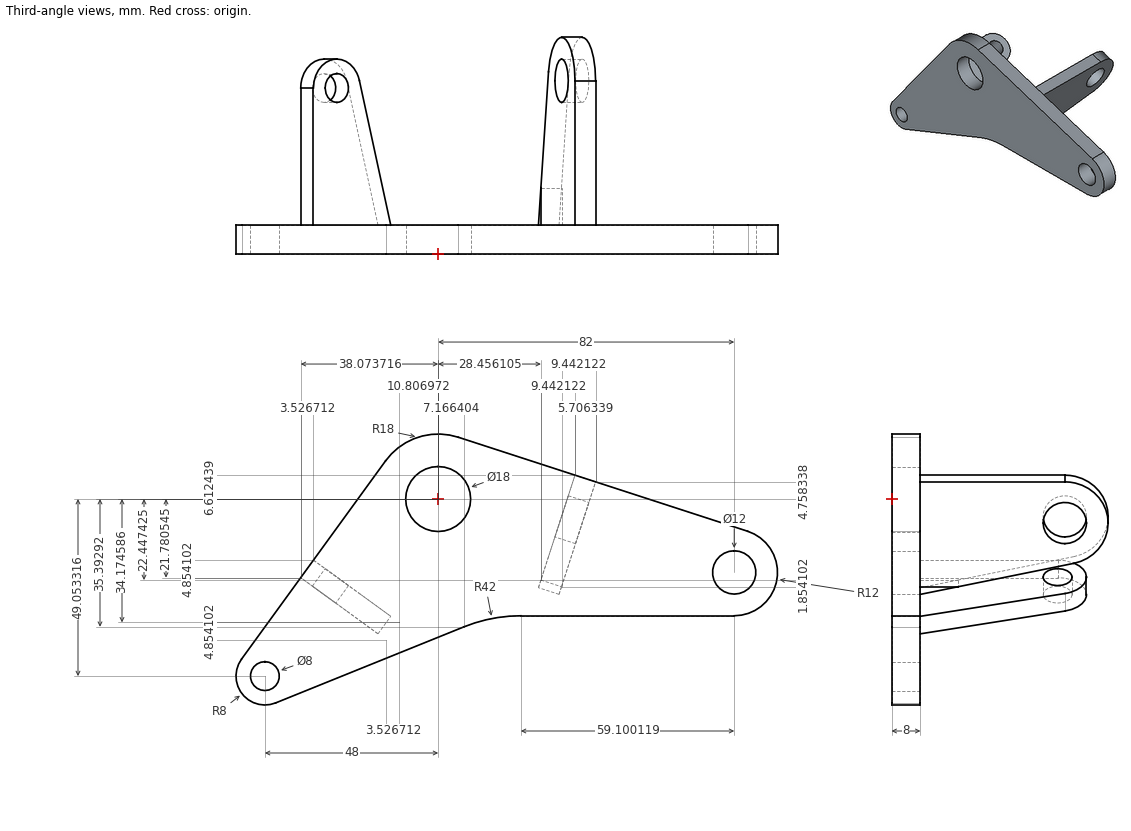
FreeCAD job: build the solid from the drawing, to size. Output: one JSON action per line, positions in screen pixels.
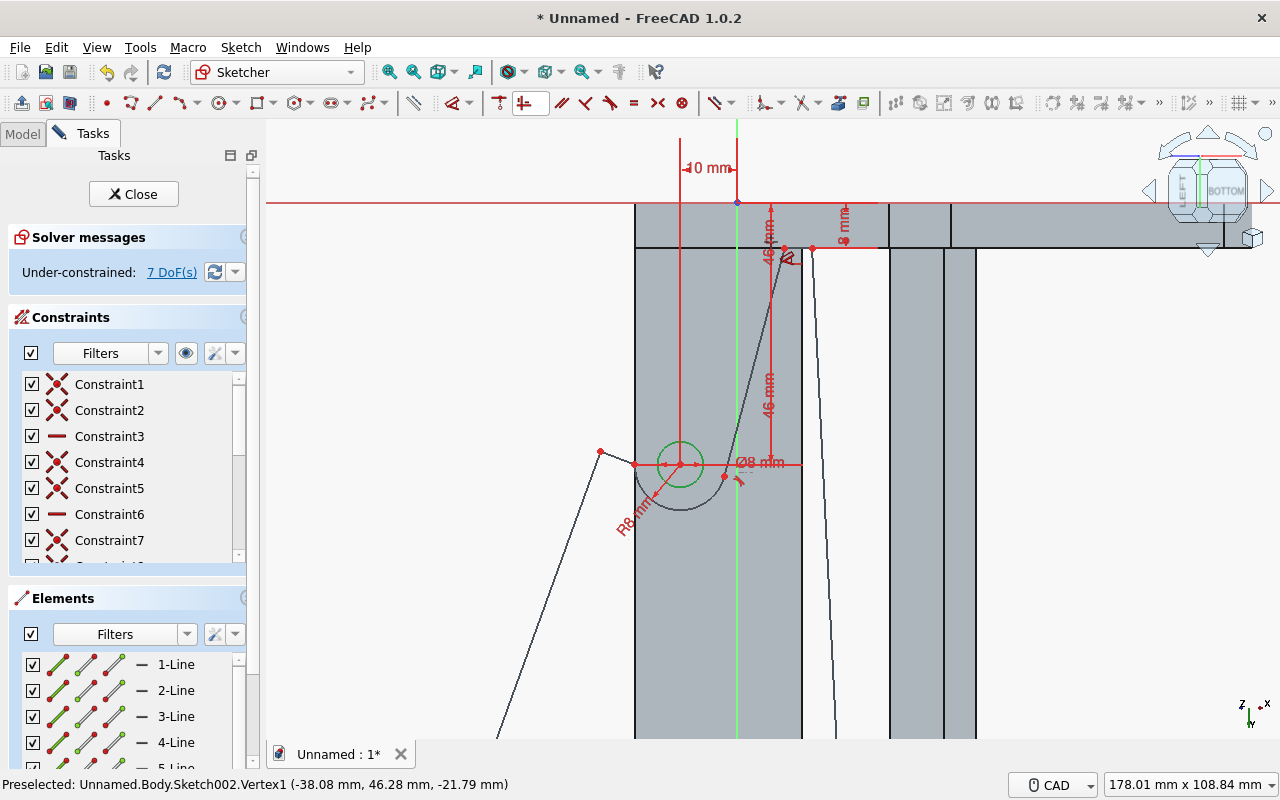
{"action": "scroll", "coordinate": [801, 248], "scroll_direction": "up", "scroll_amount": 2}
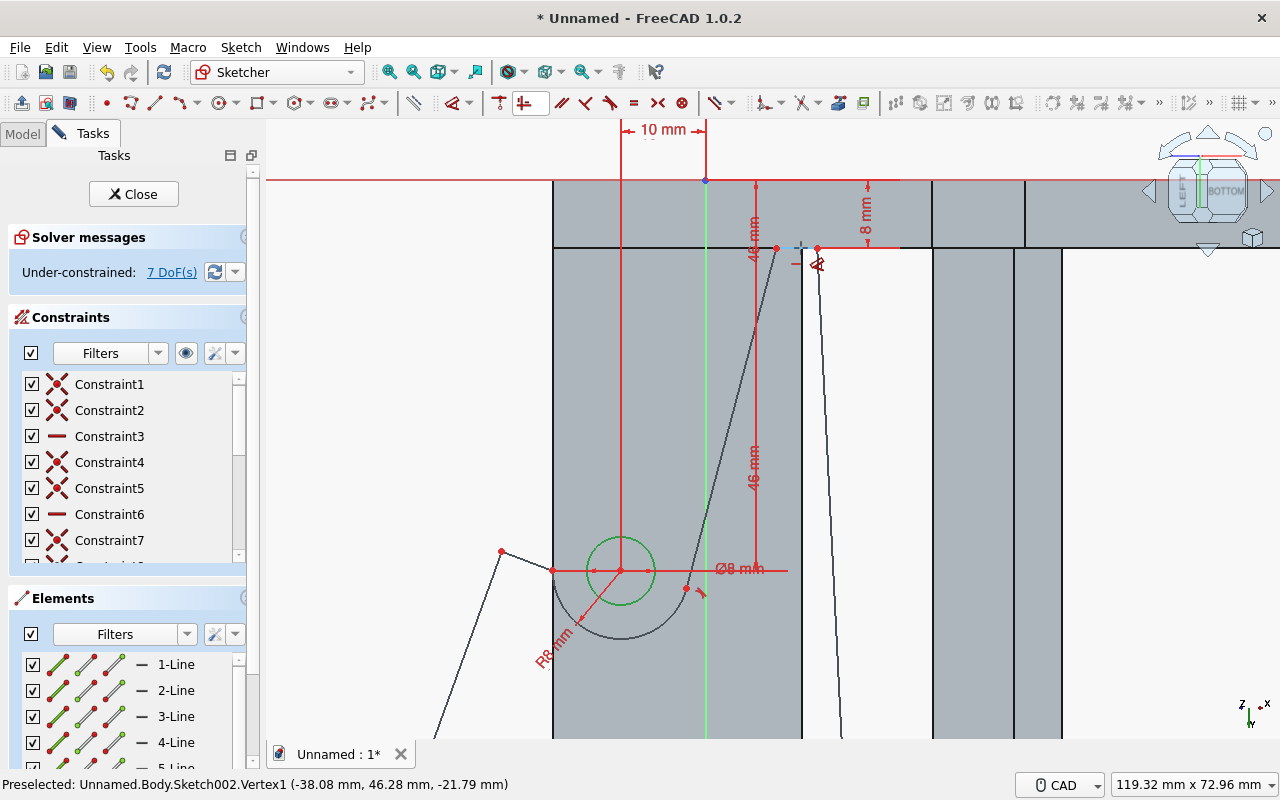
{"action": "left_click", "coordinate": [801, 248]}
{"action": "left_click", "coordinate": [797, 214]}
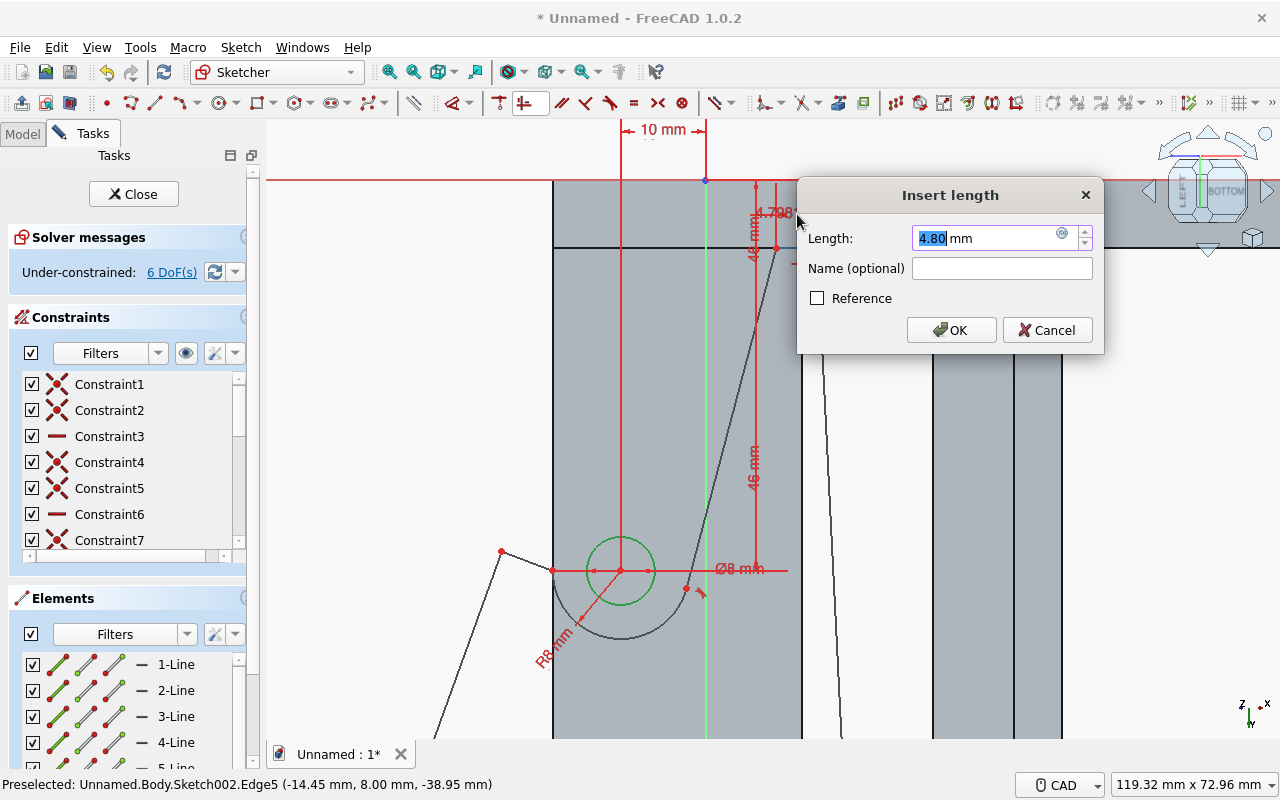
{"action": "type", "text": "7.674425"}
{"action": "key", "text": "Return"}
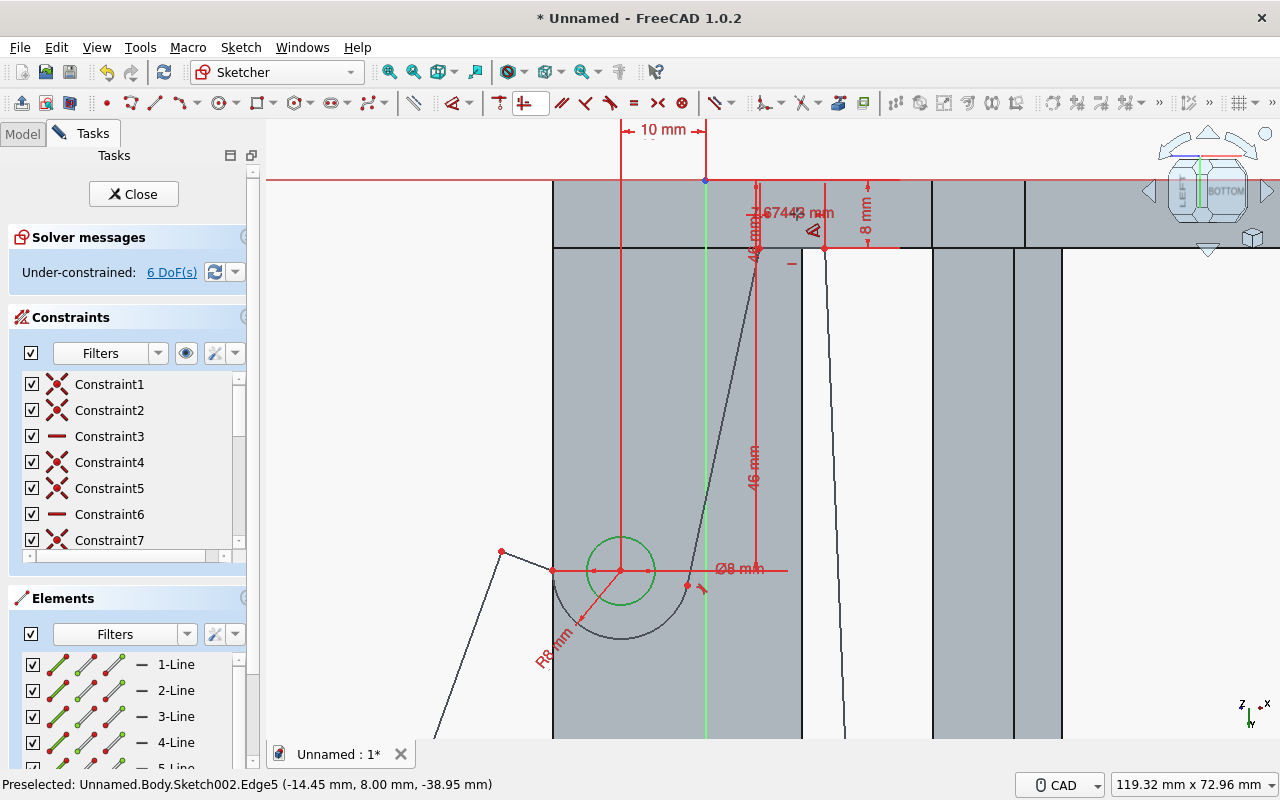
{"action": "left_click", "coordinate": [538, 565]}
{"action": "left_click", "coordinate": [527, 518]}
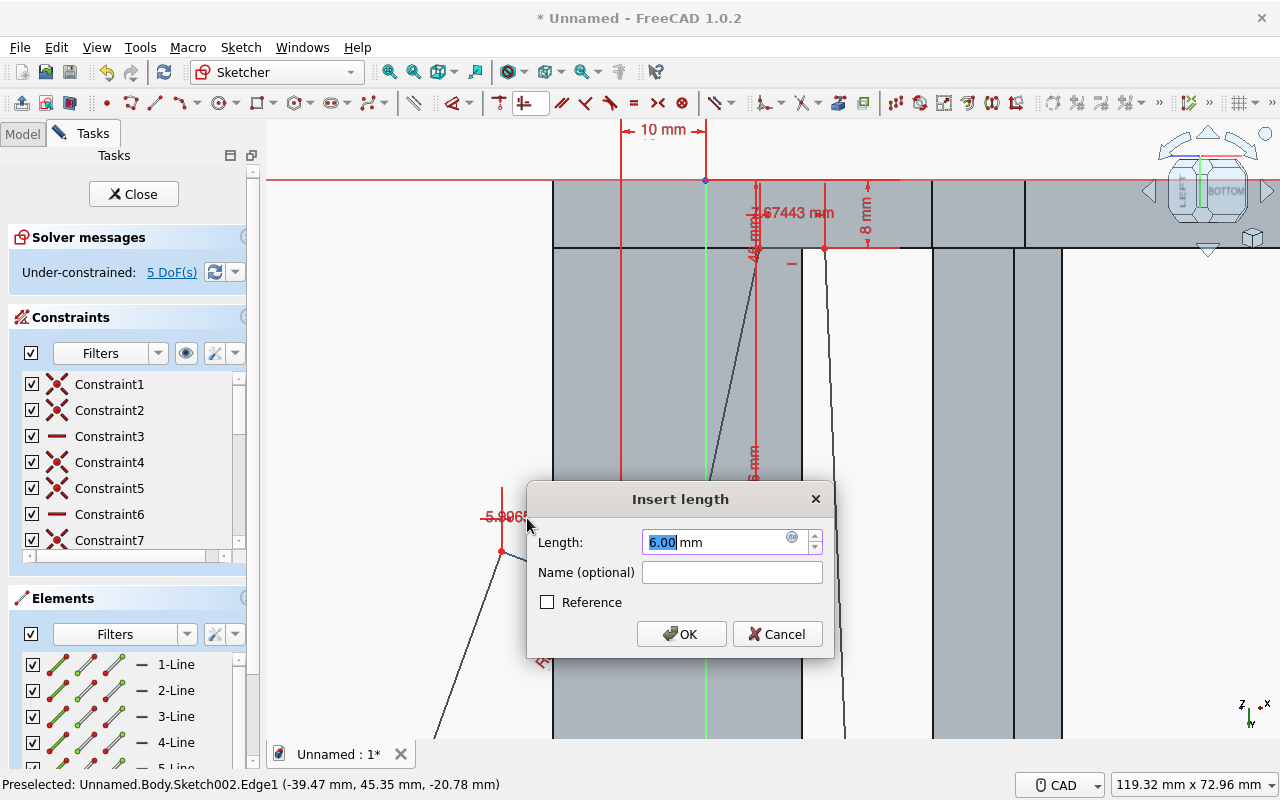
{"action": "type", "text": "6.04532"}
{"action": "key", "text": "Return"}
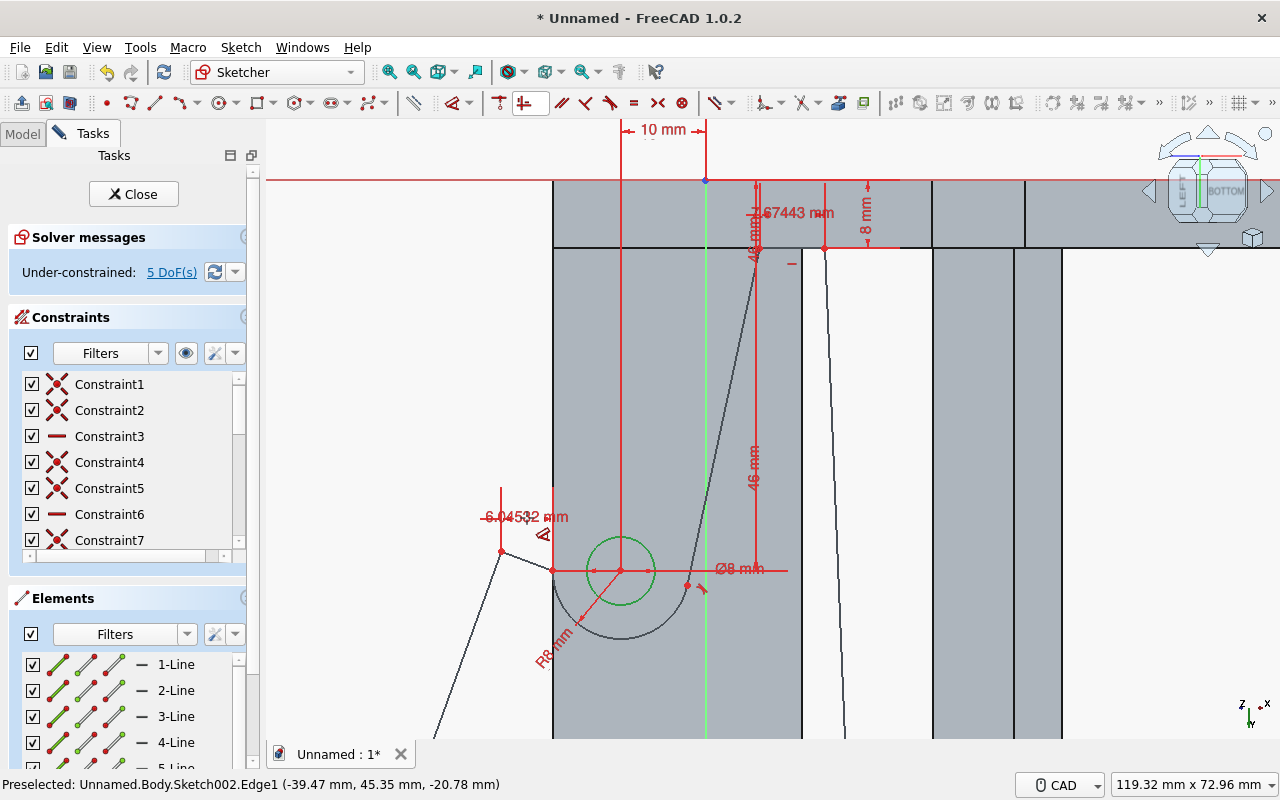
{"action": "scroll", "coordinate": [808, 249], "scroll_direction": "down", "scroll_amount": 4}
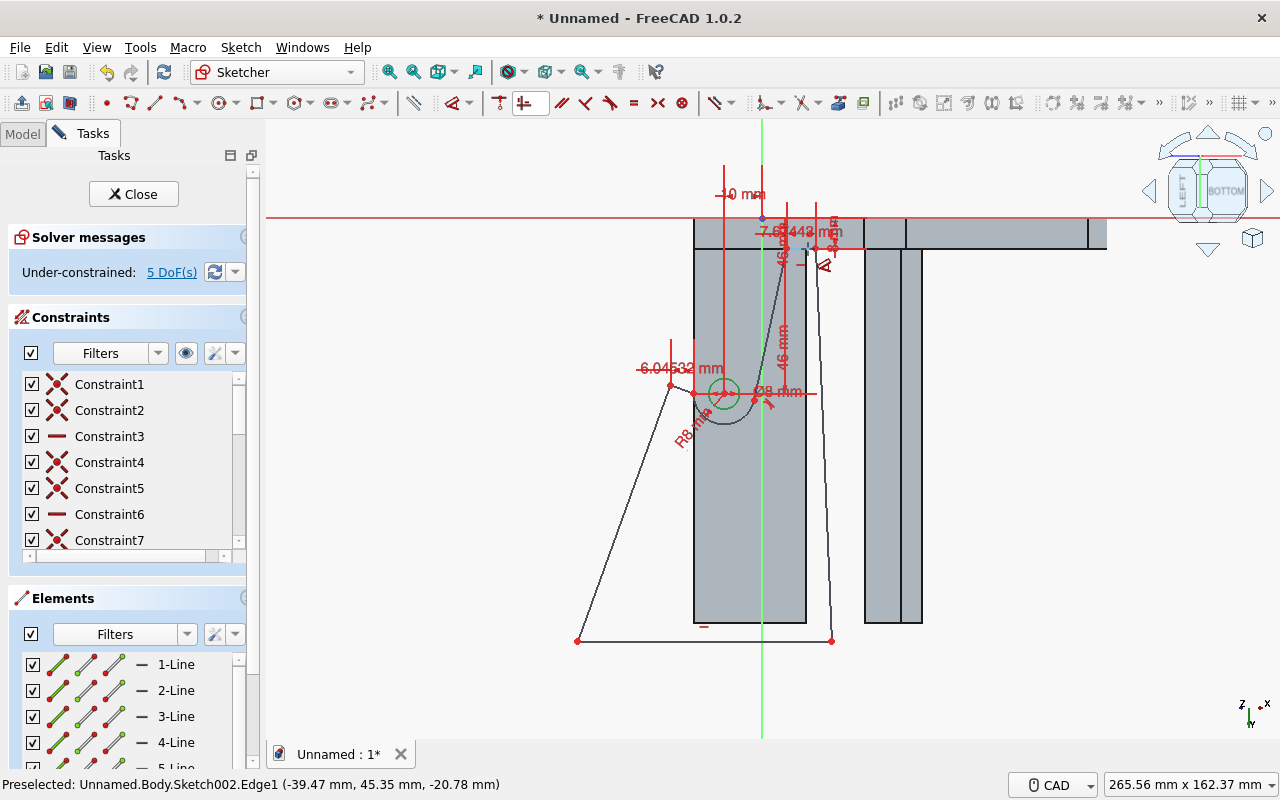
{"action": "left_click", "coordinate": [654, 642]}
{"action": "left_click", "coordinate": [705, 676]}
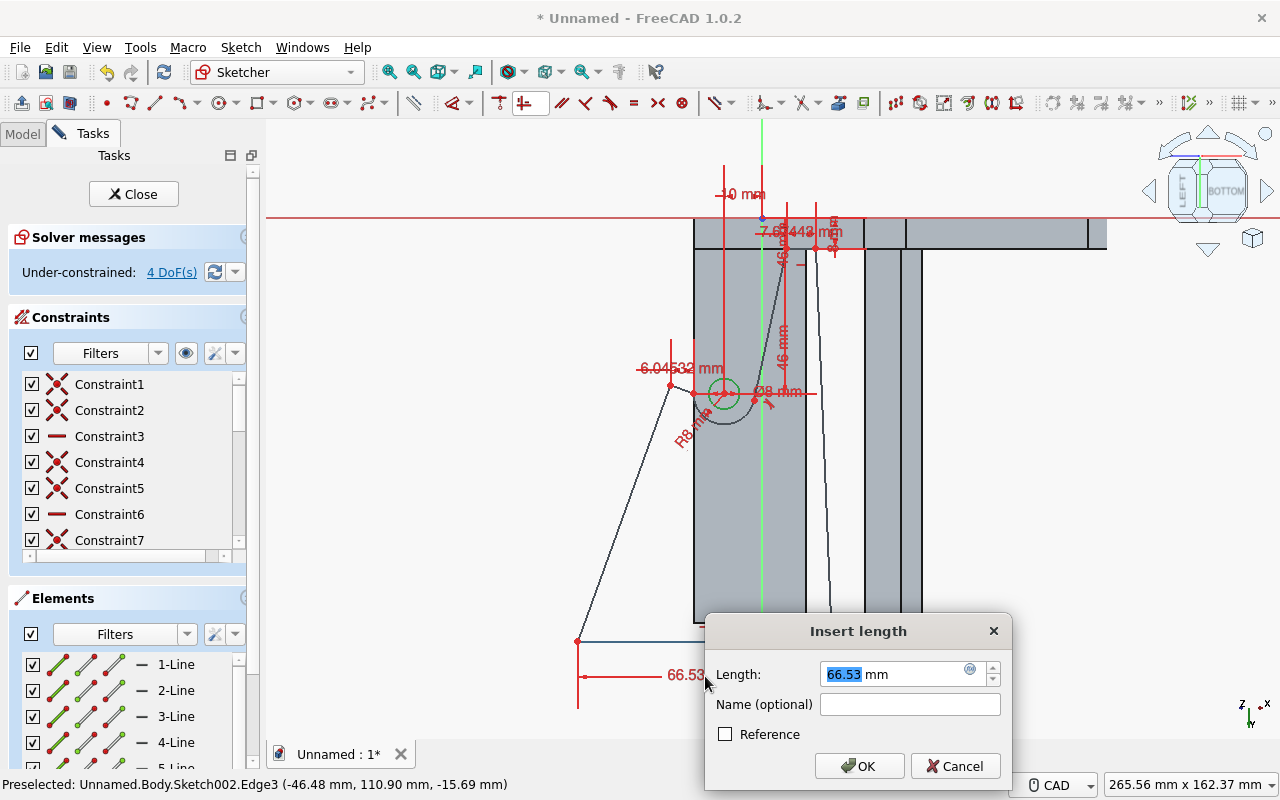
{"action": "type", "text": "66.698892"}
{"action": "key", "text": "Return"}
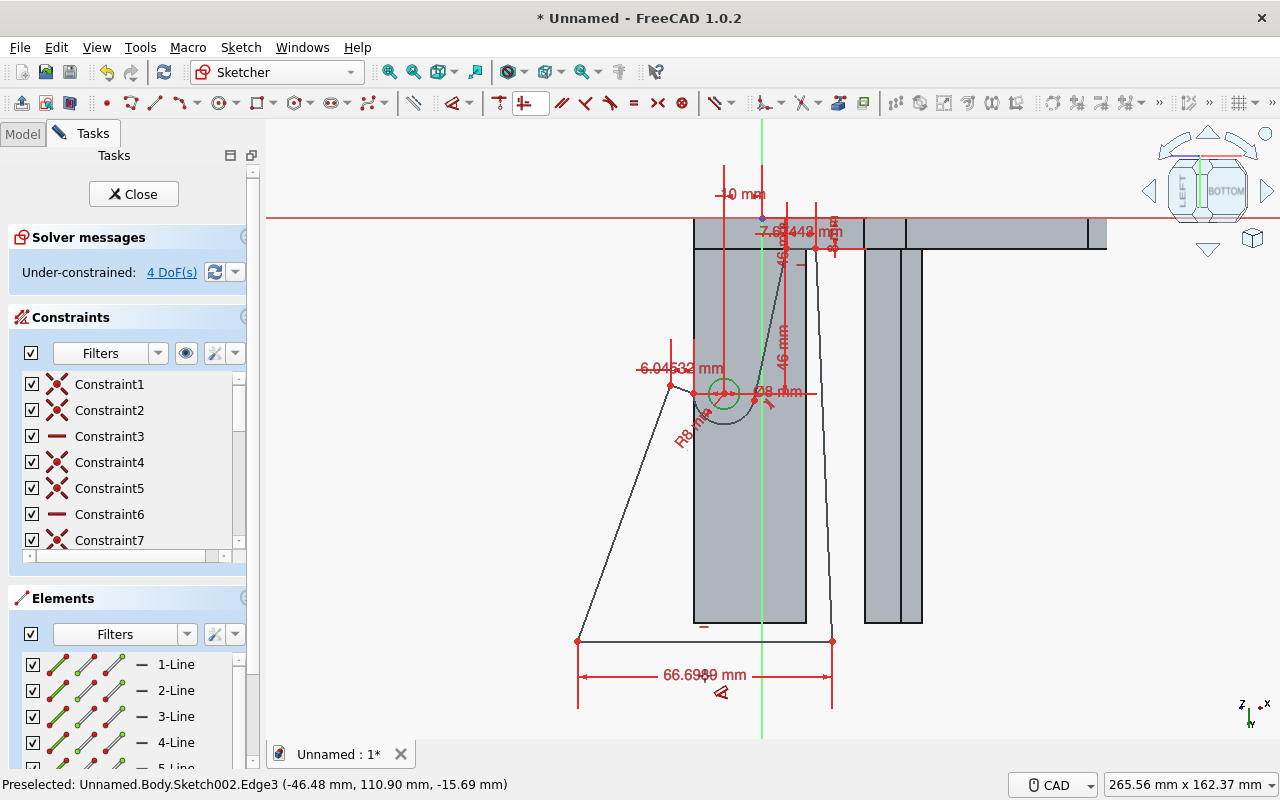
{"action": "scroll", "coordinate": [787, 249], "scroll_direction": "up", "scroll_amount": 2}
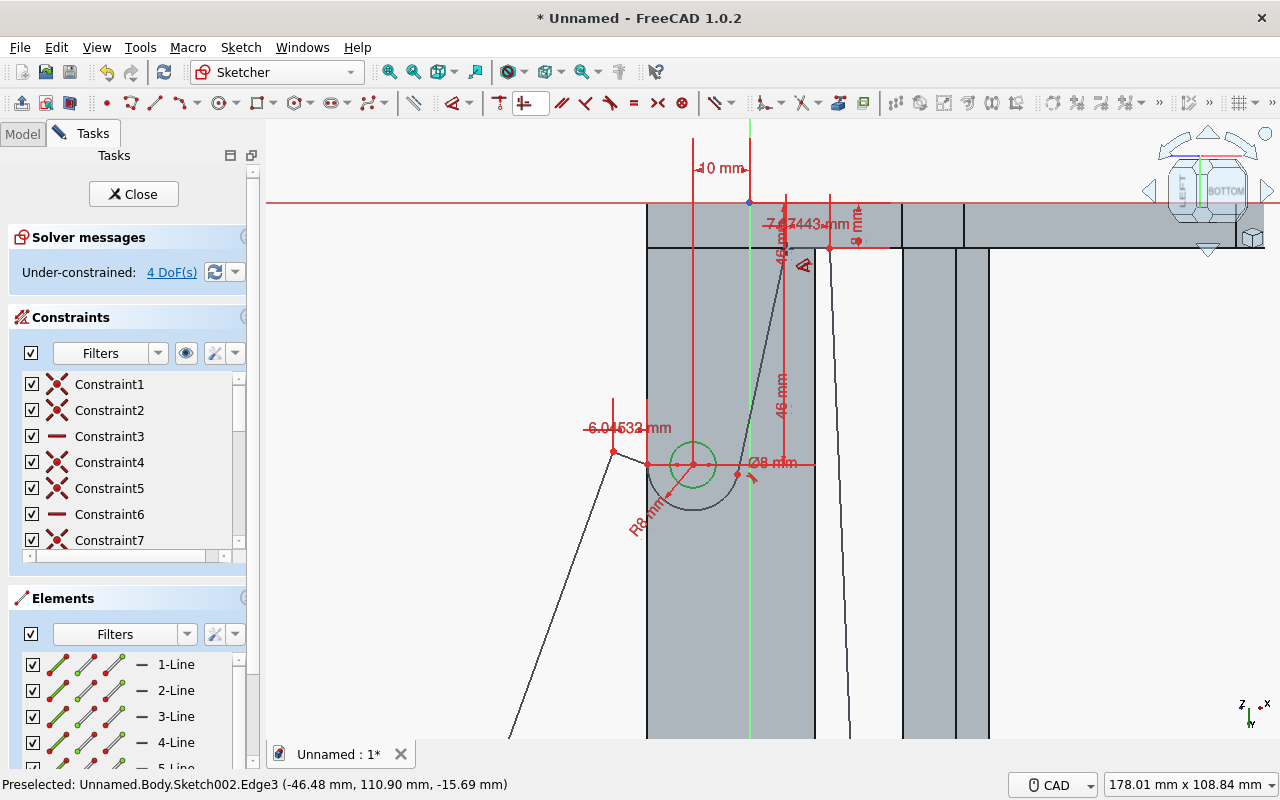
{"action": "left_click", "coordinate": [786, 248]}
{"action": "left_click", "coordinate": [781, 354]}